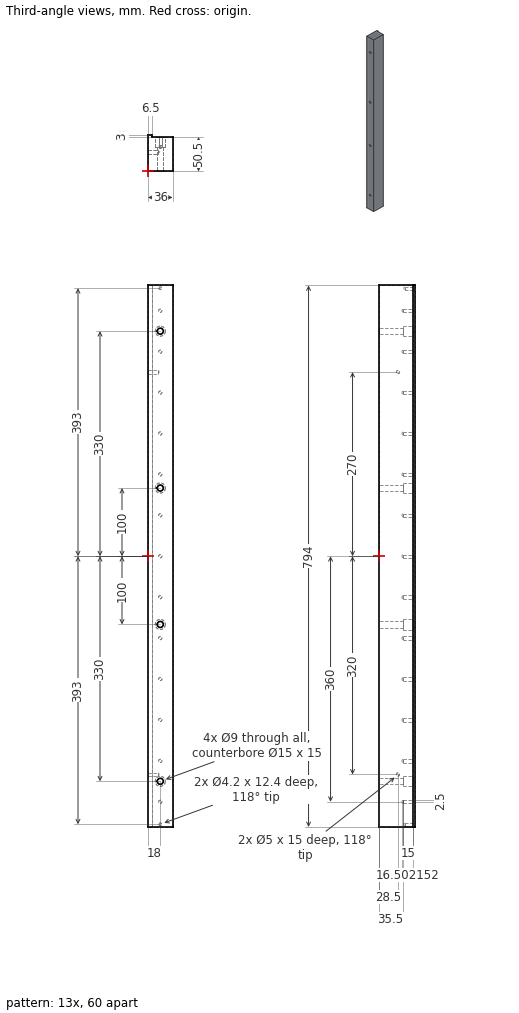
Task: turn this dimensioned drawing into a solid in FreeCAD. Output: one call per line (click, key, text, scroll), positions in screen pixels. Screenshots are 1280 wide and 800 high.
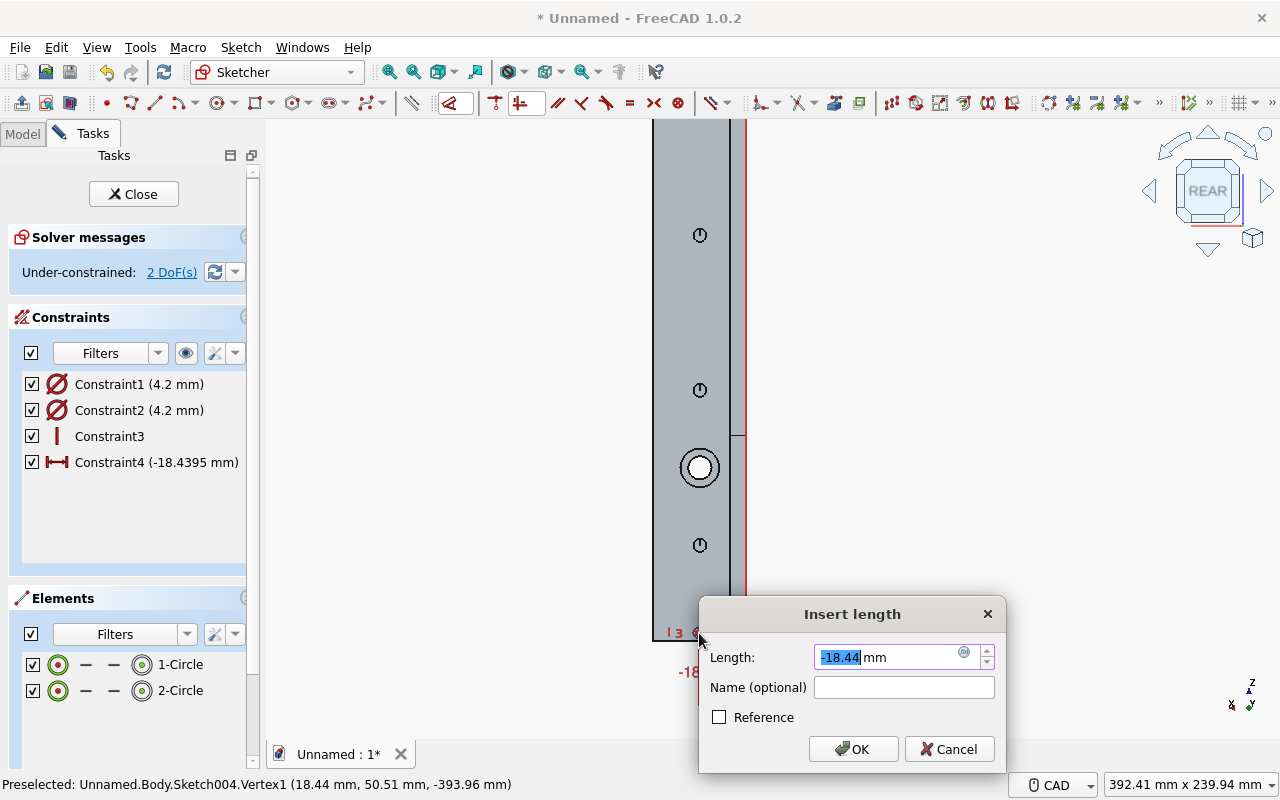
text(-18)
key(Return)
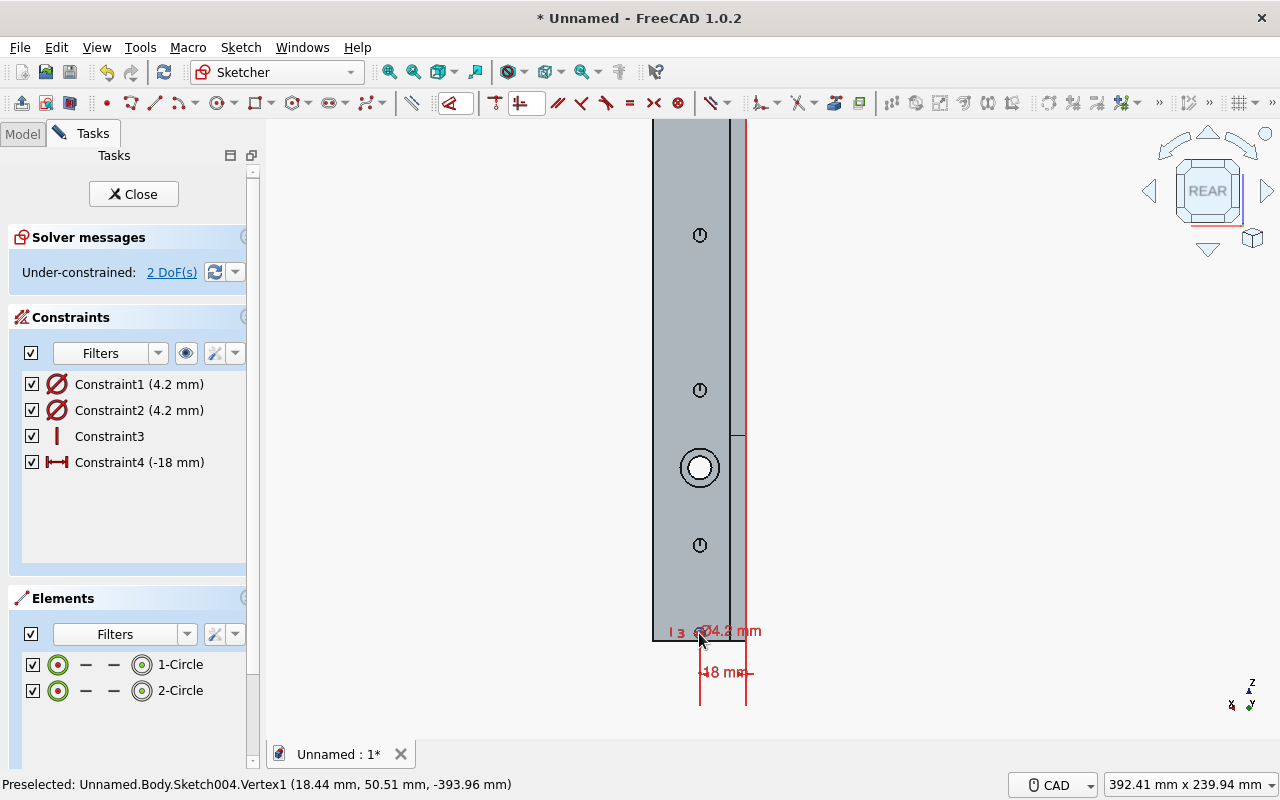
scroll(700, 635, down, 8)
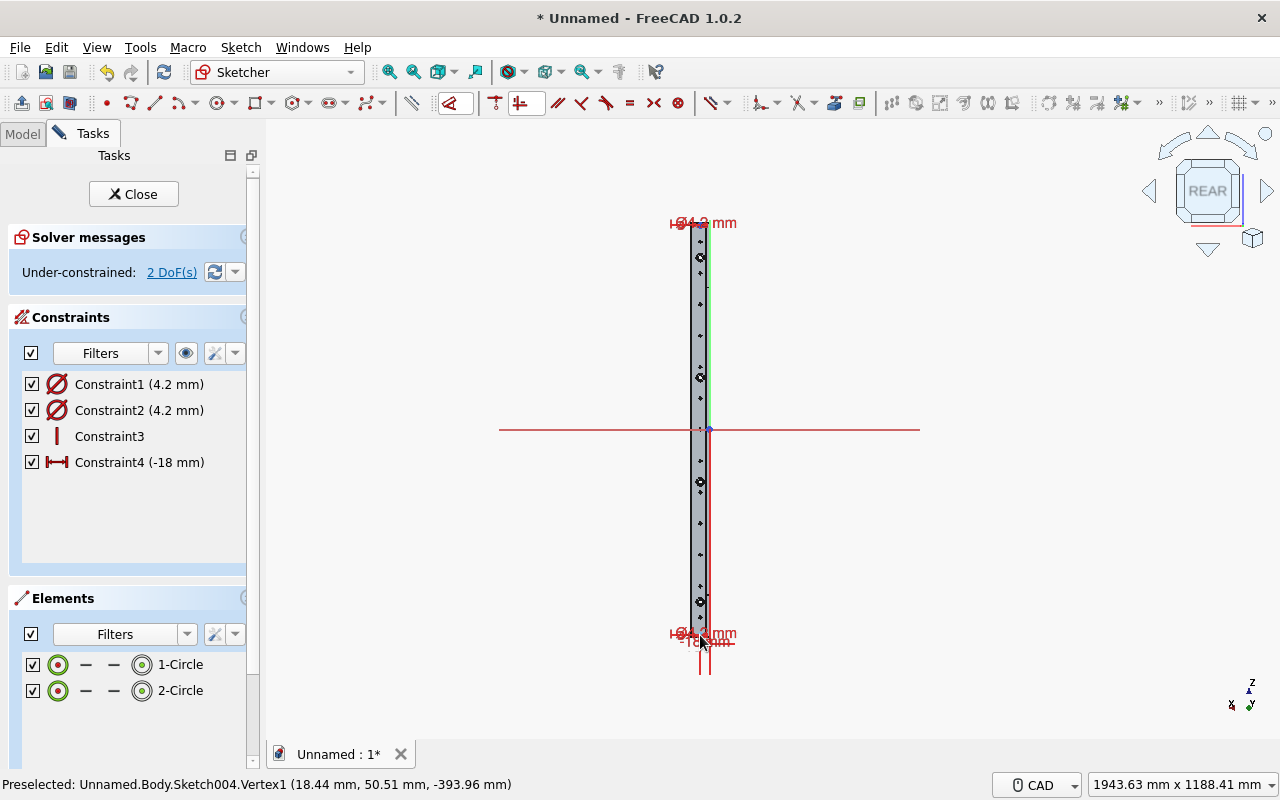
click(700, 635)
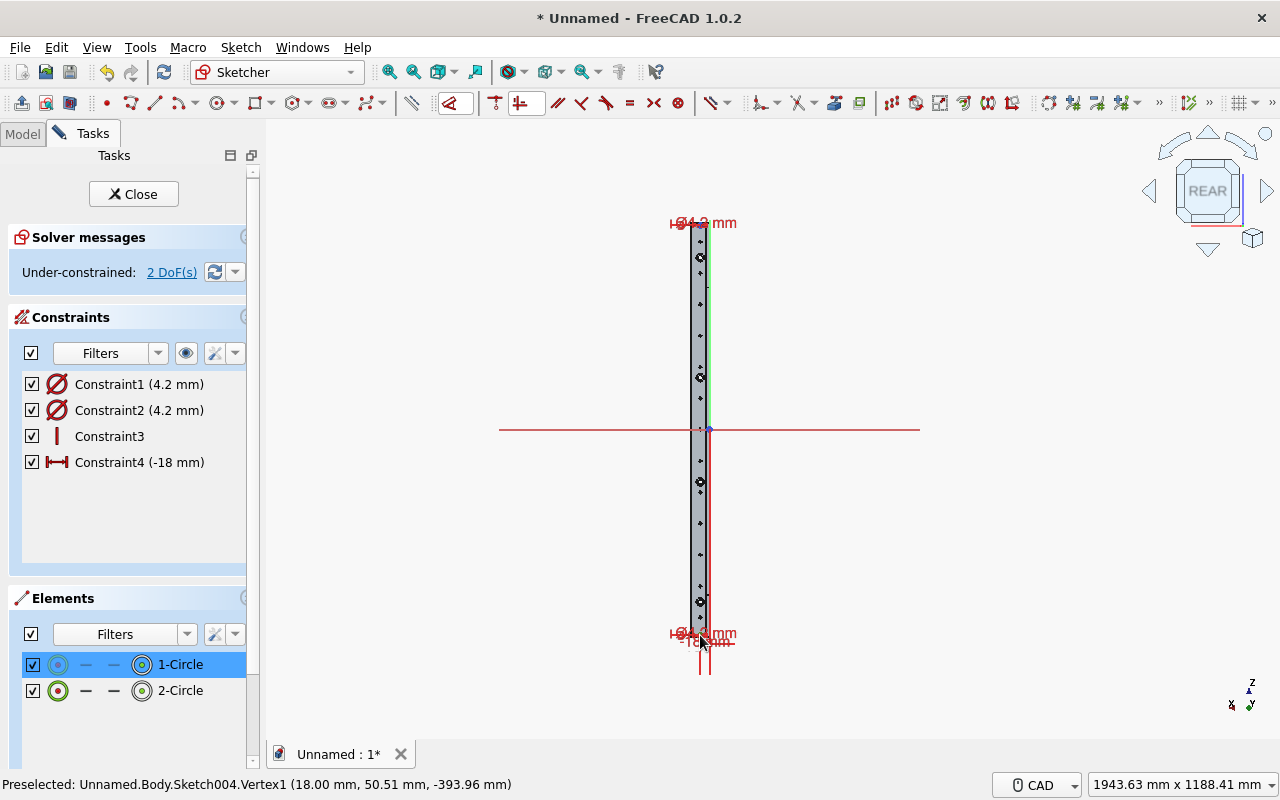
click(468, 104)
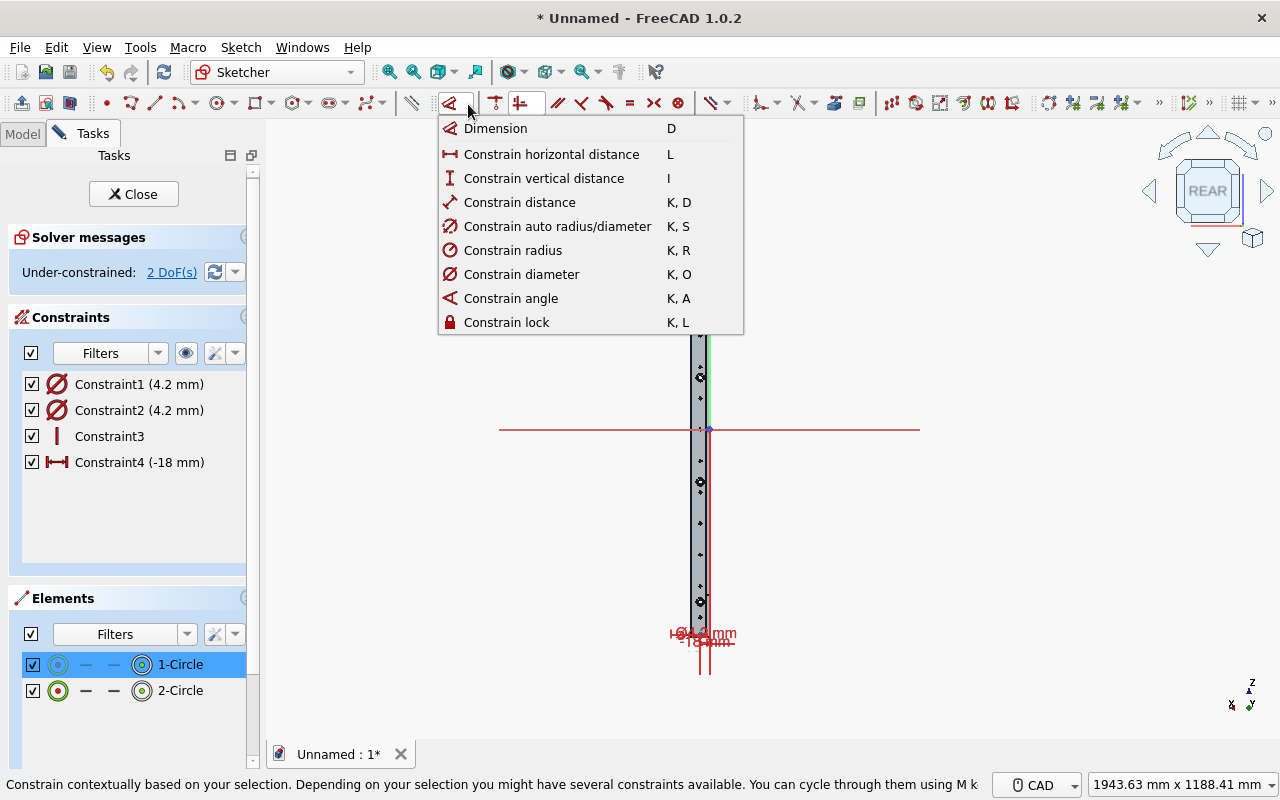
click(591, 178)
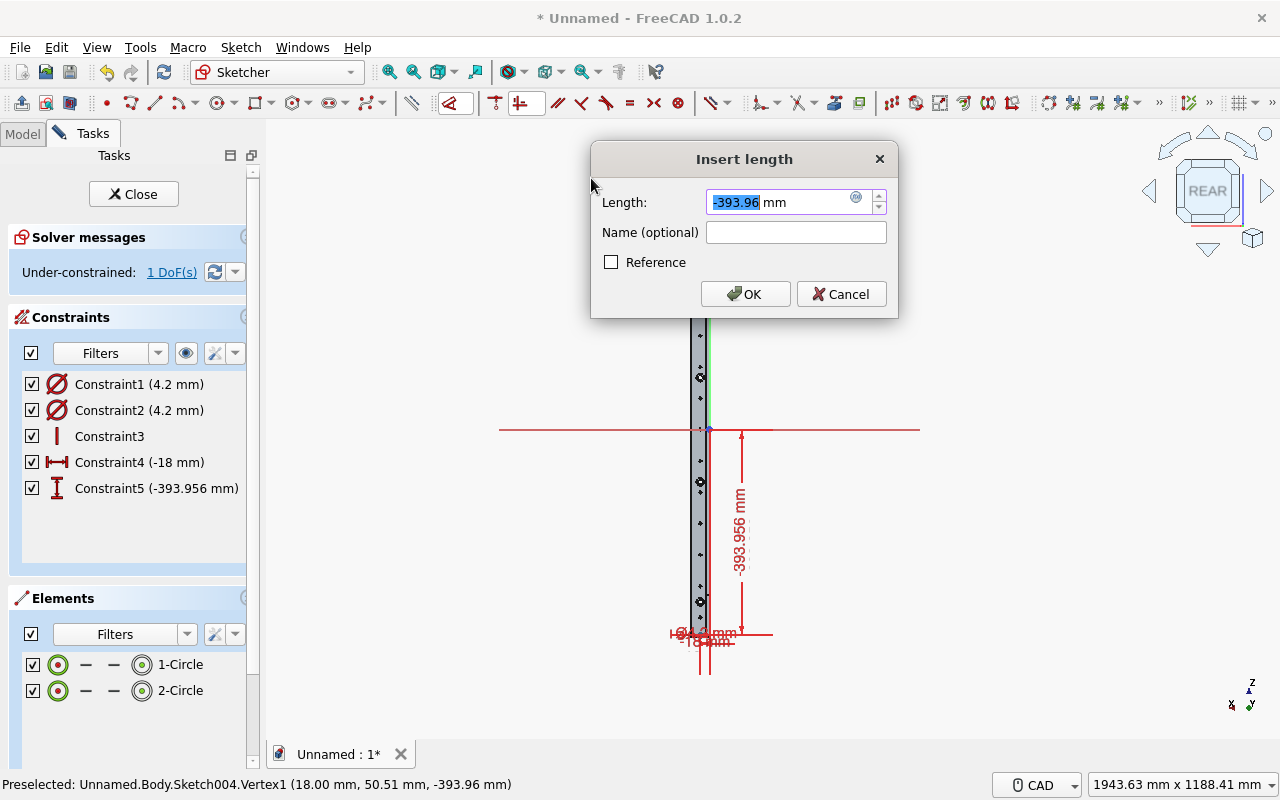
text(-393)
key(Return)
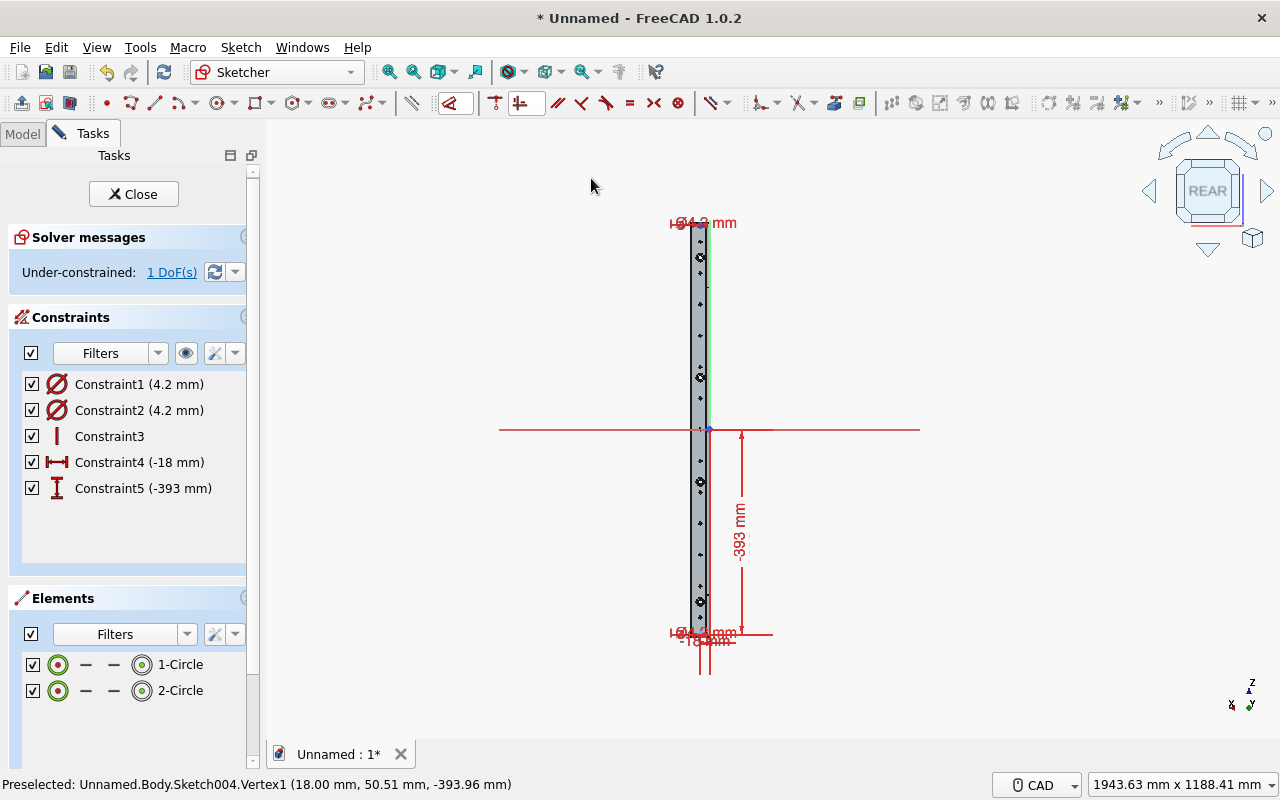
click(700, 225)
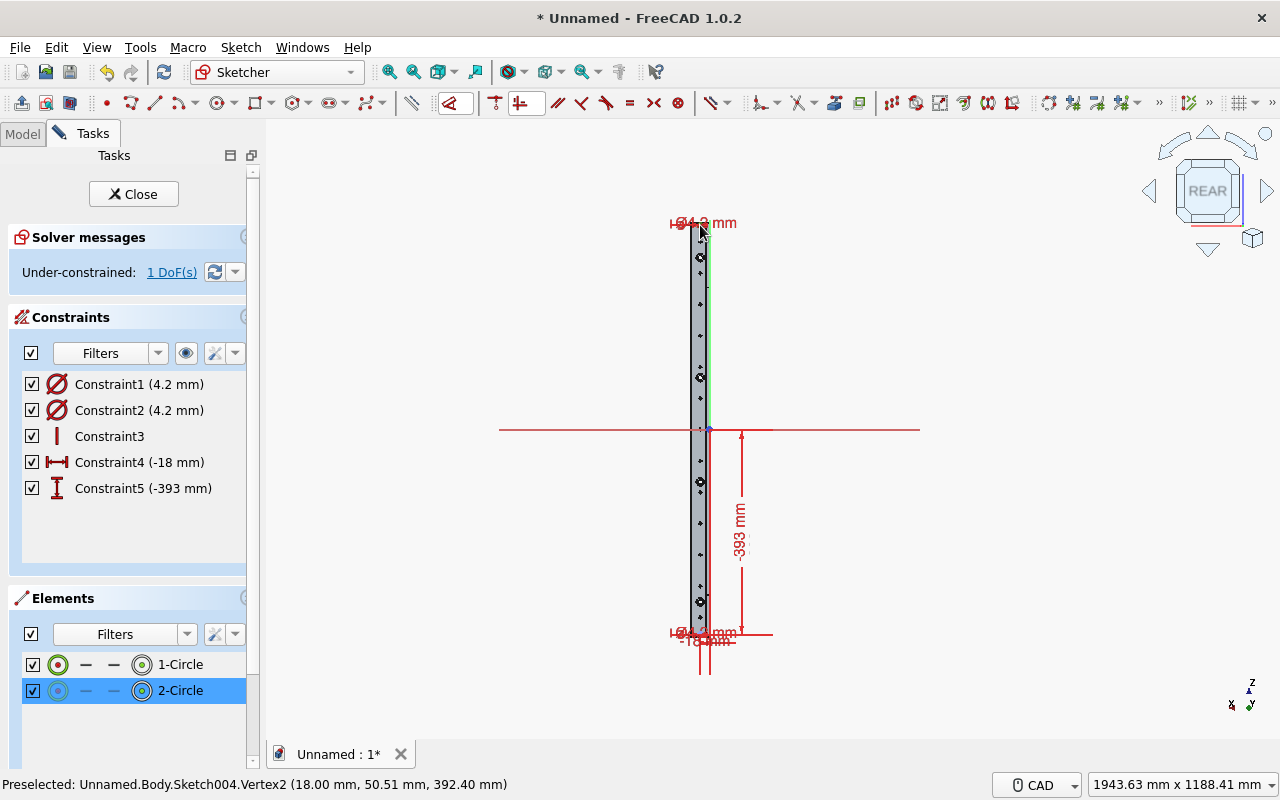
click(468, 104)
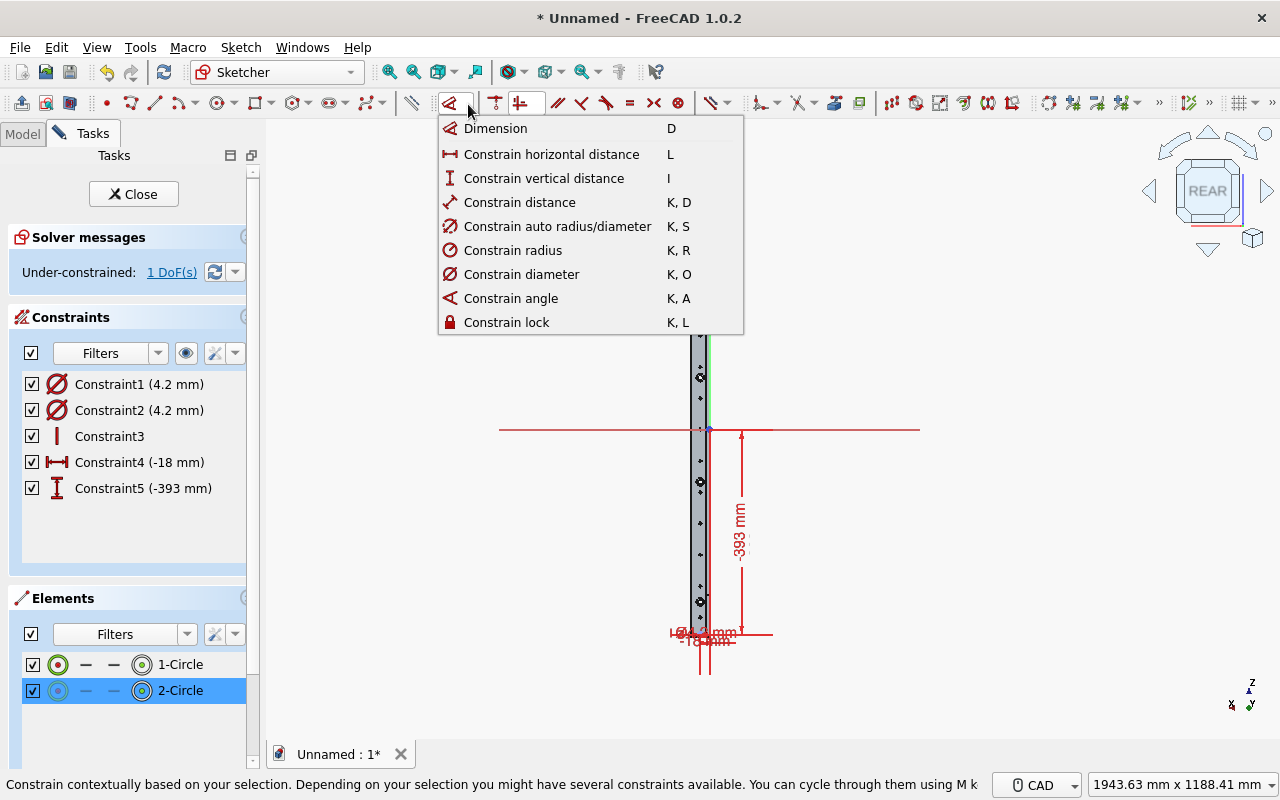
click(591, 178)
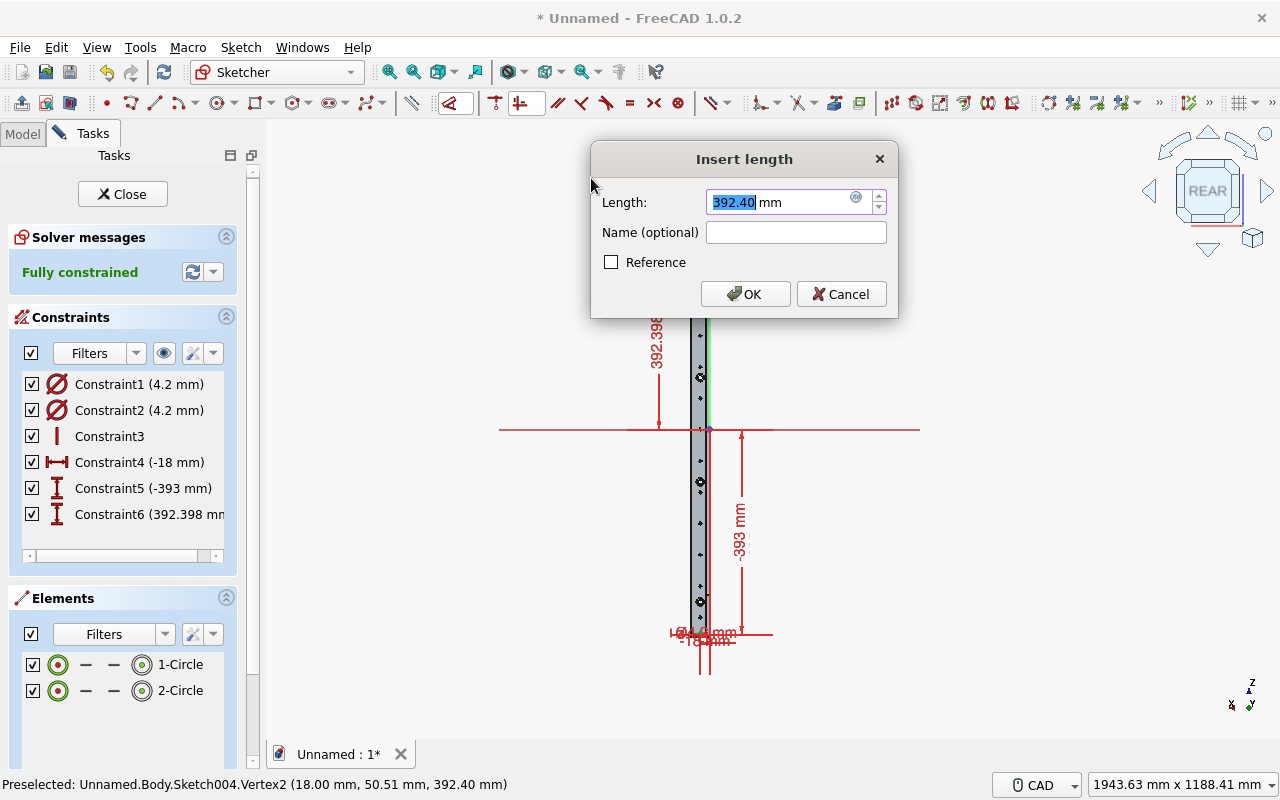
text(393)
key(Return)